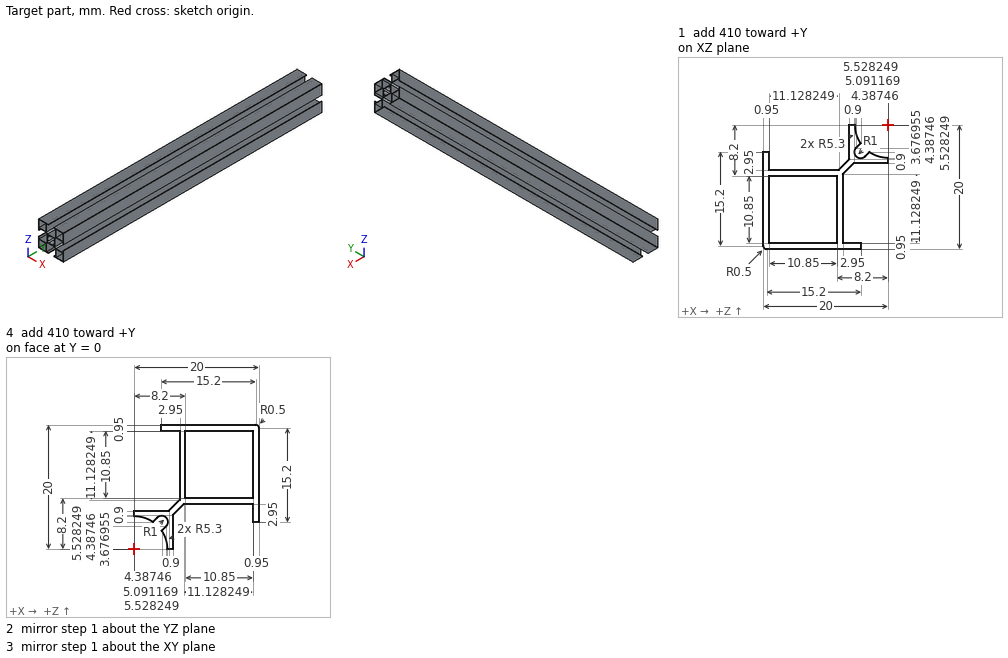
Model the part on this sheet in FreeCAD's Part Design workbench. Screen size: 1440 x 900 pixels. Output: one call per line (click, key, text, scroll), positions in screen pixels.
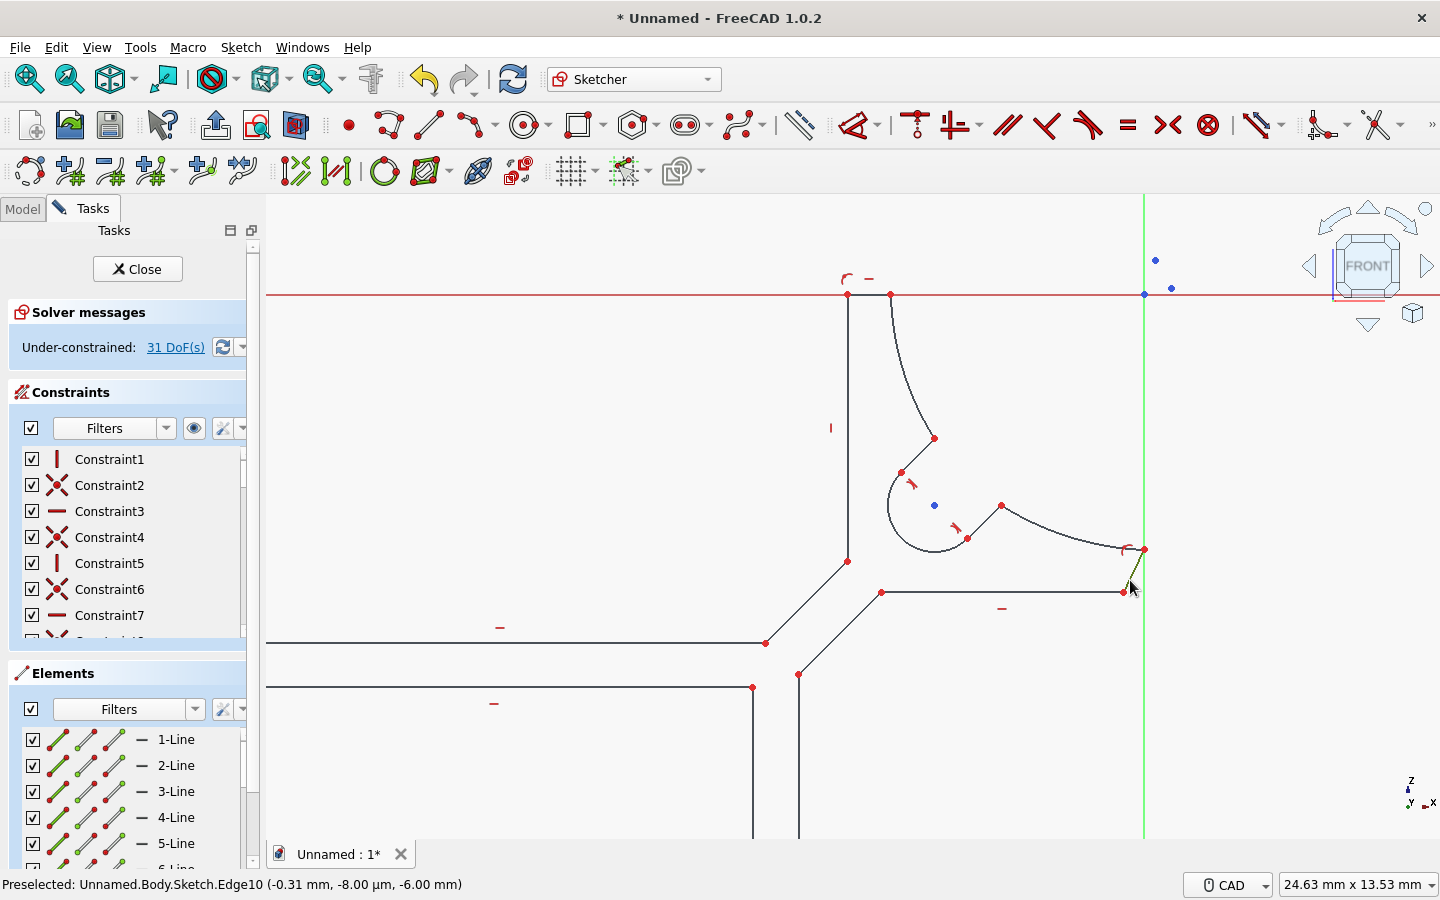
click(982, 126)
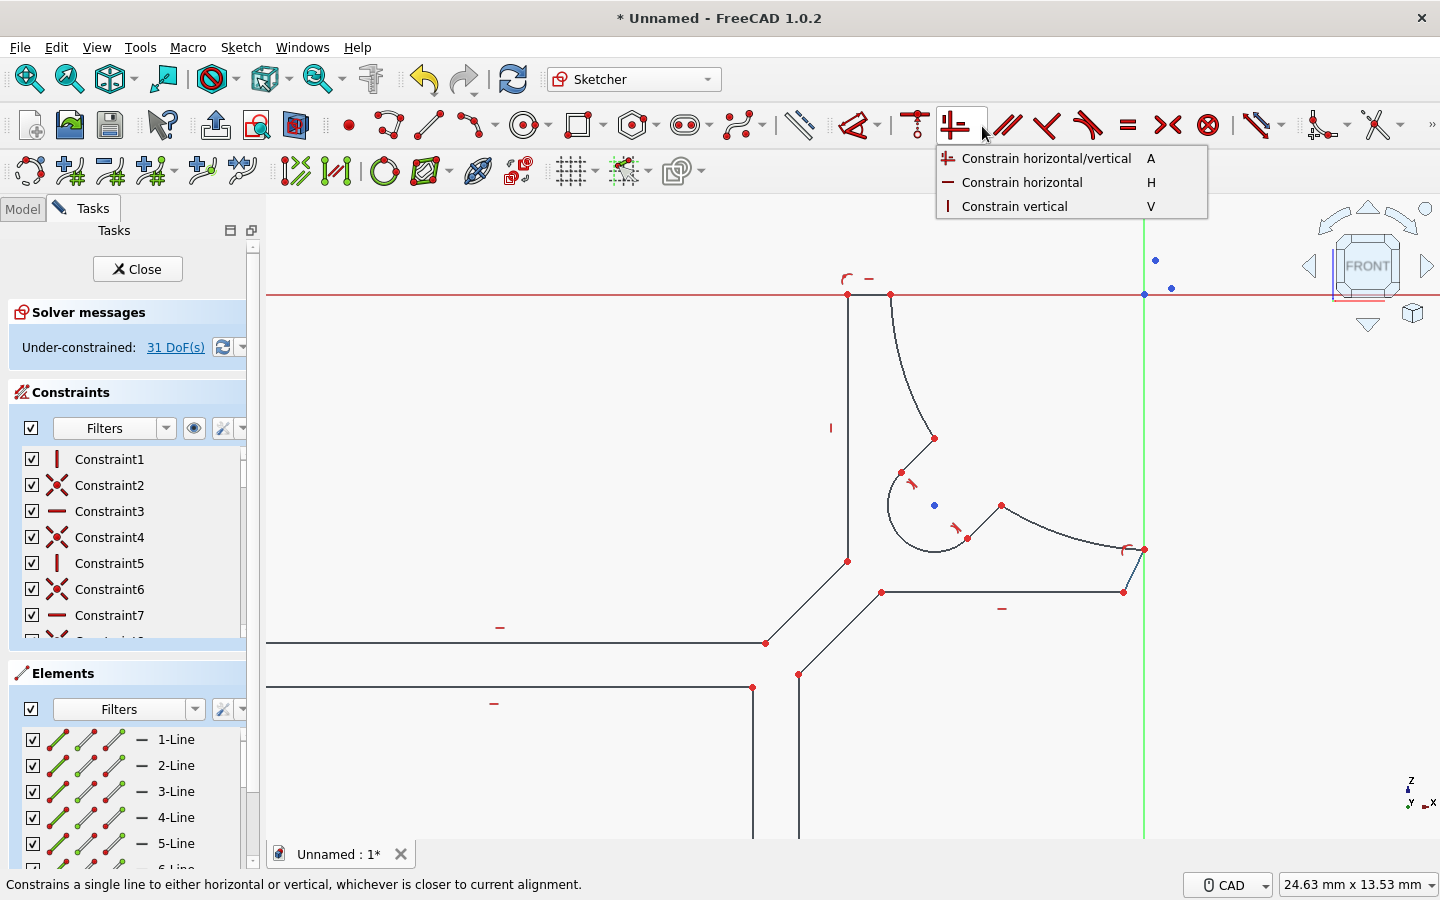
click(1072, 206)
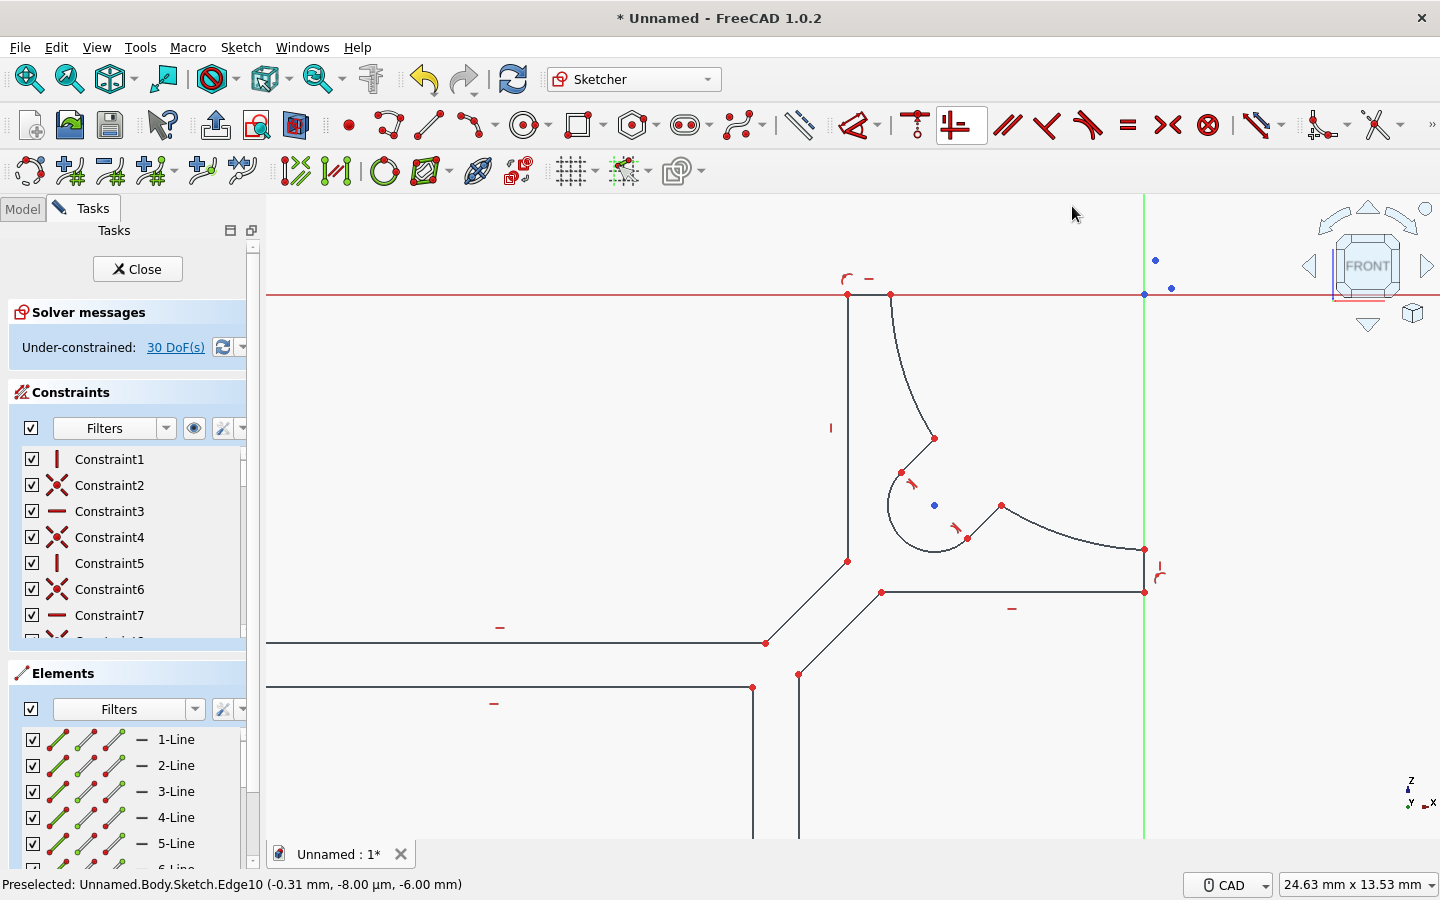
click(896, 340)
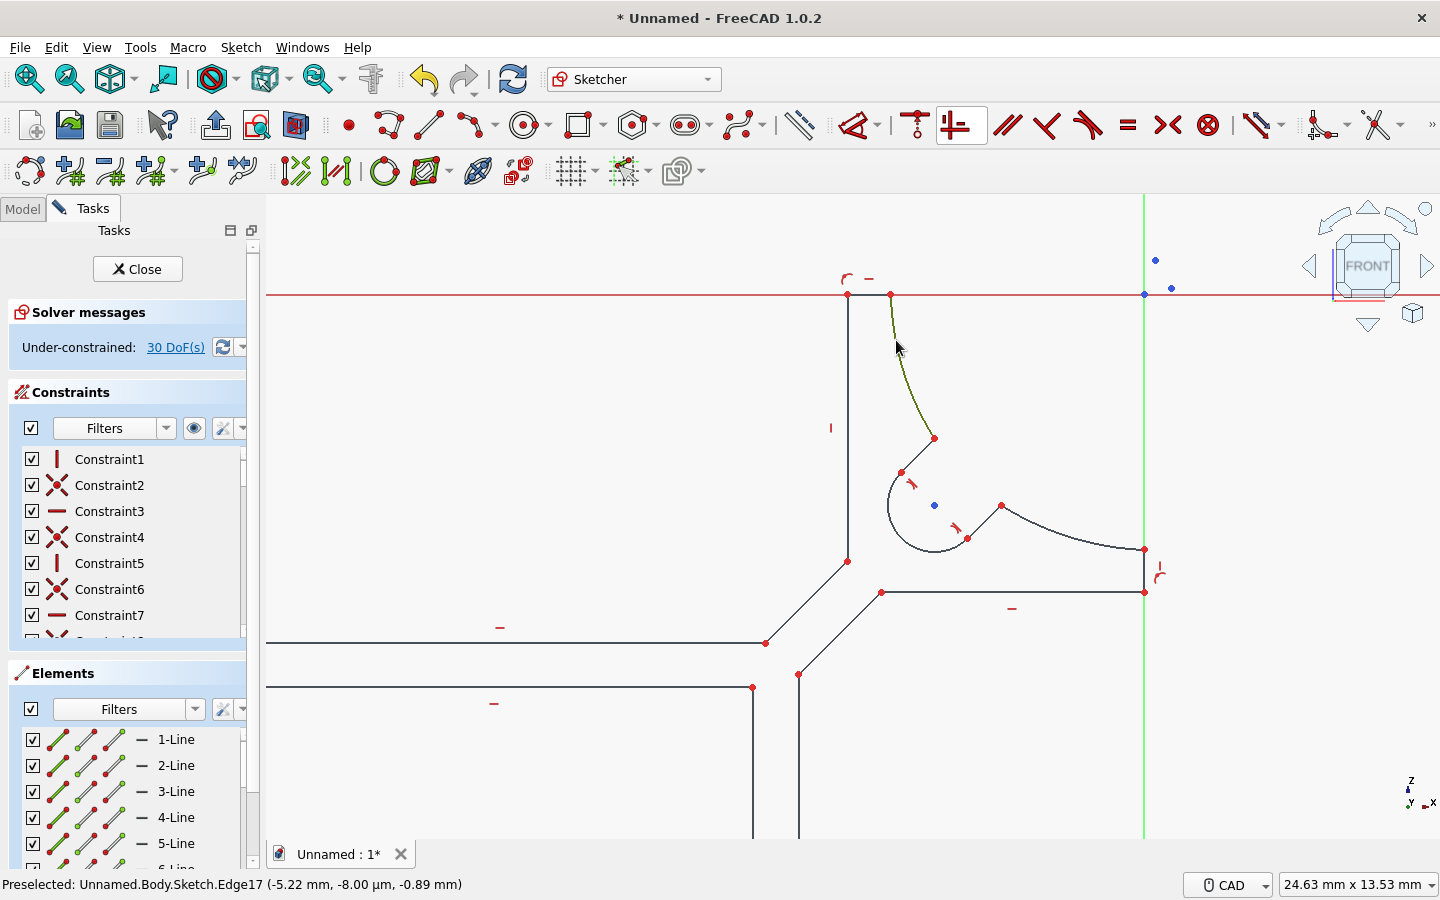
click(1041, 527)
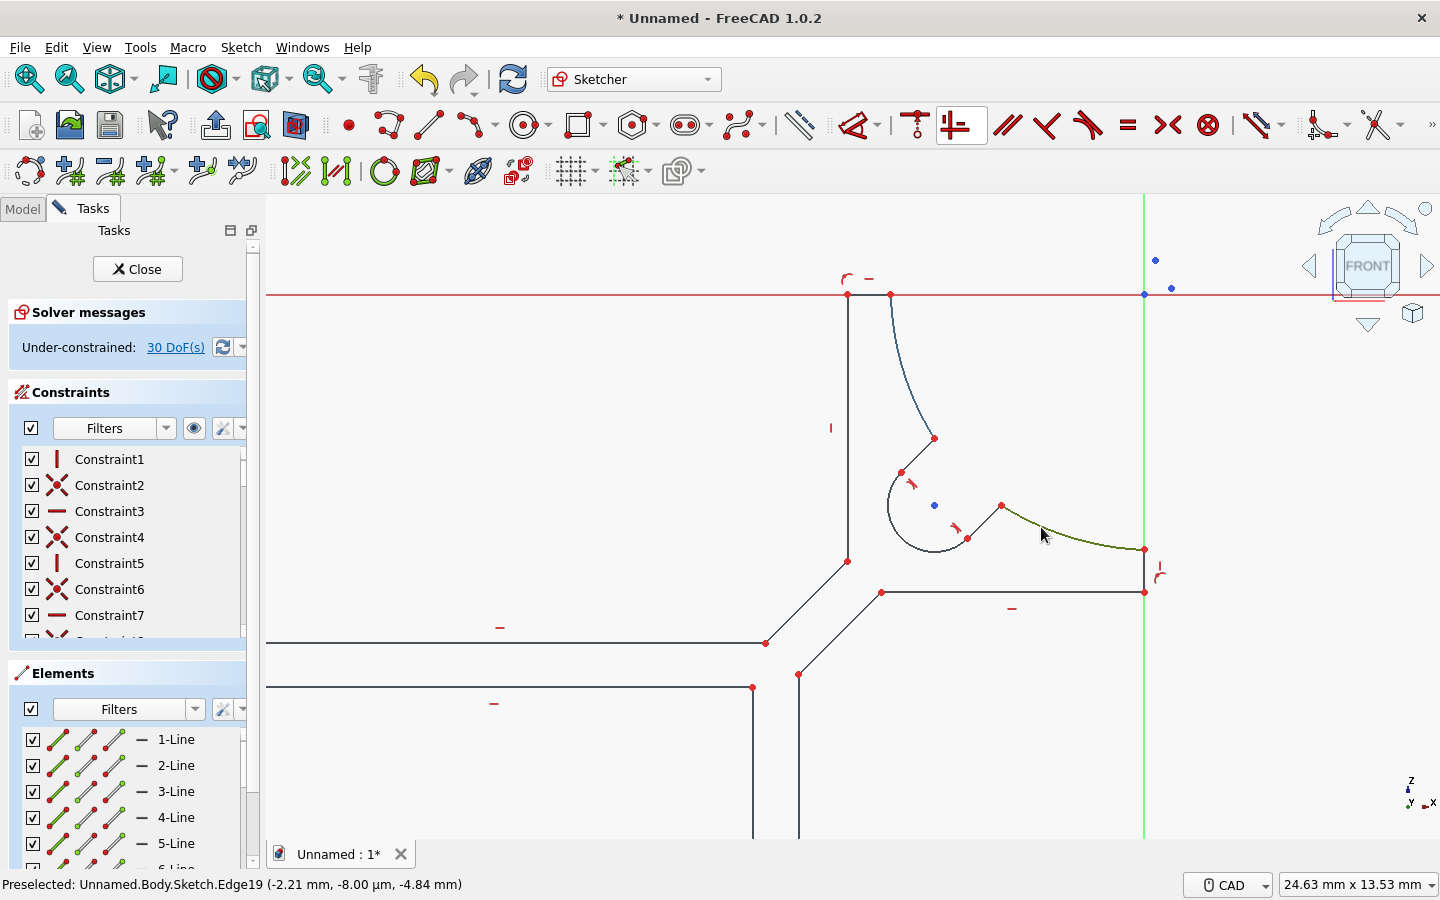
click(916, 126)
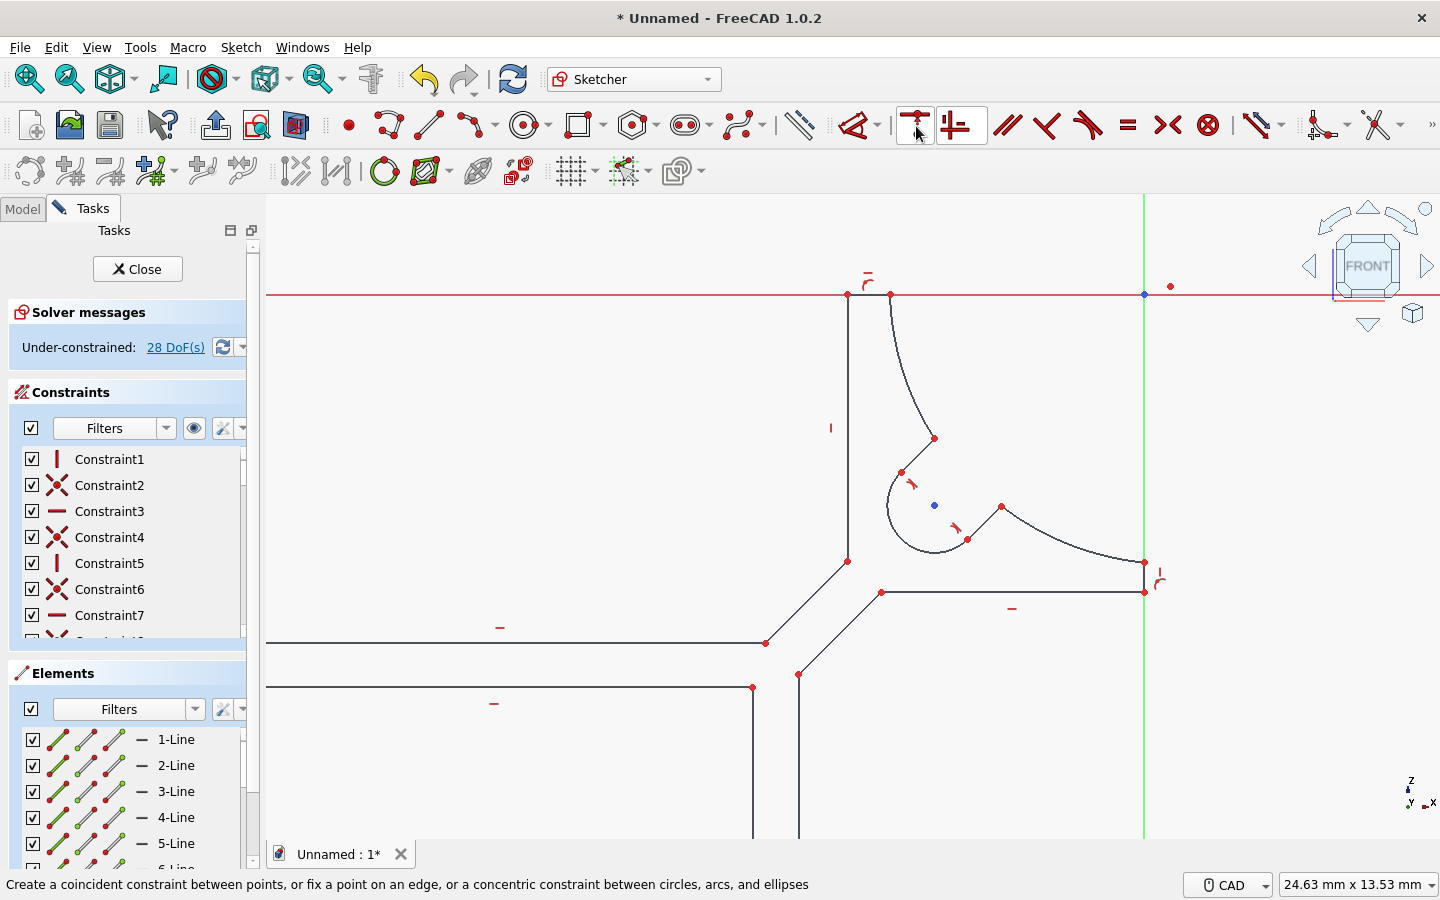
scroll(1157, 291, up, 2)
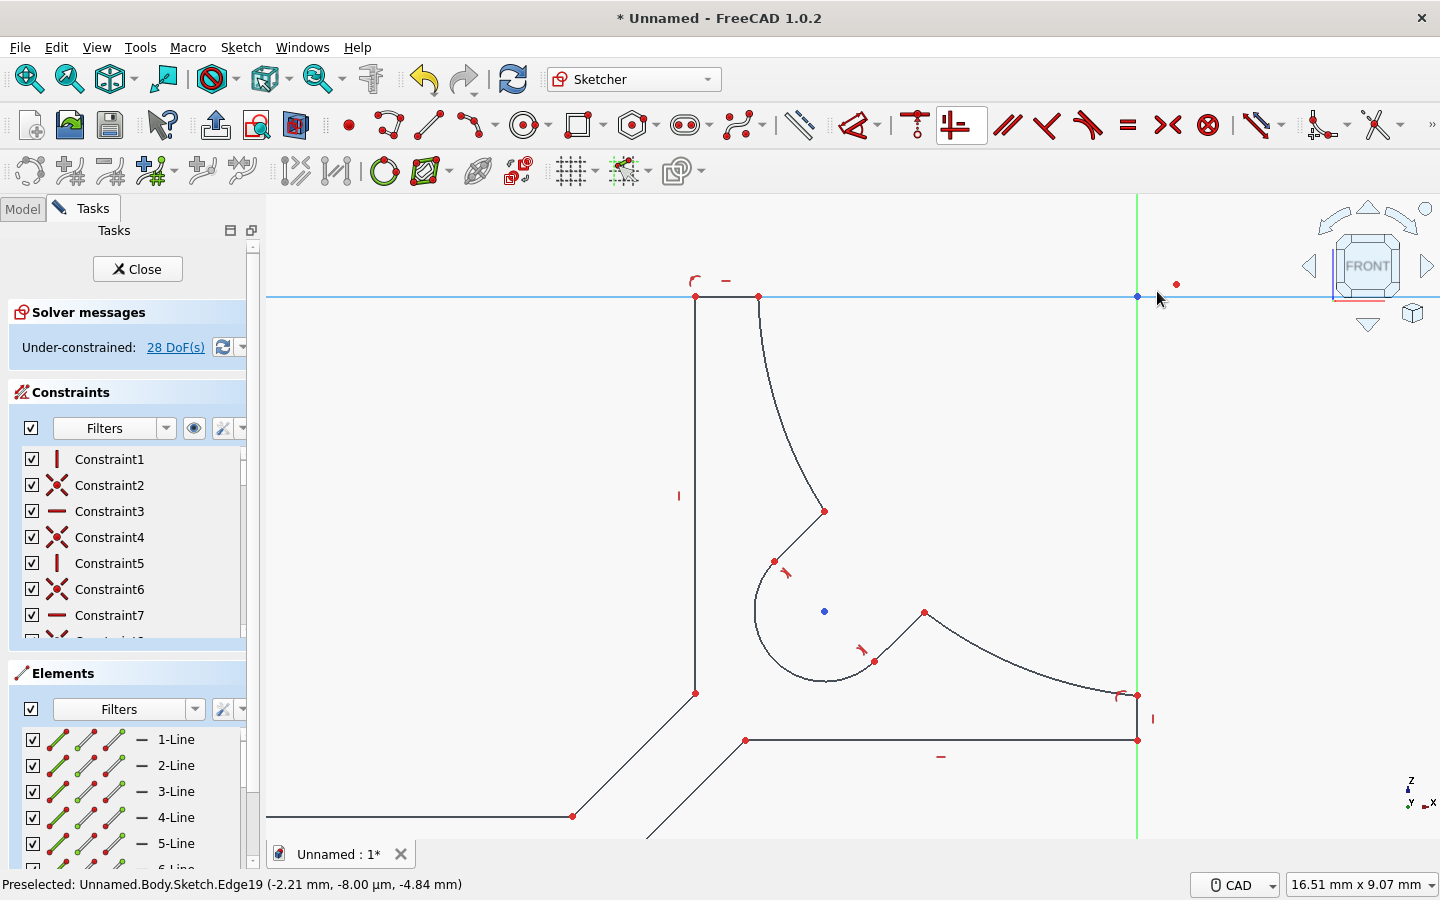
drag(1127, 275, 1187, 307)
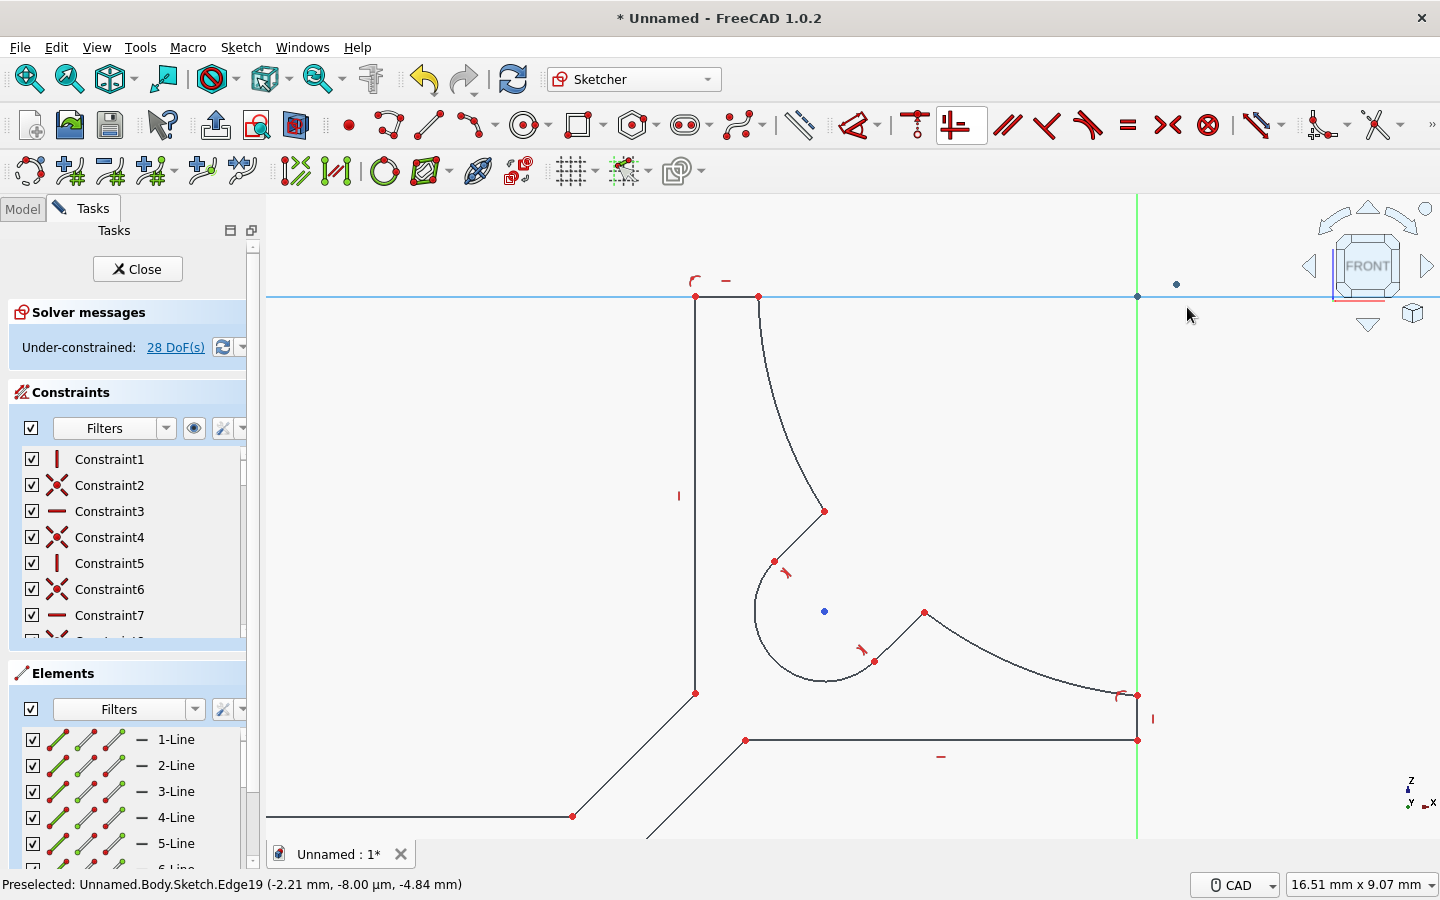
click(916, 126)